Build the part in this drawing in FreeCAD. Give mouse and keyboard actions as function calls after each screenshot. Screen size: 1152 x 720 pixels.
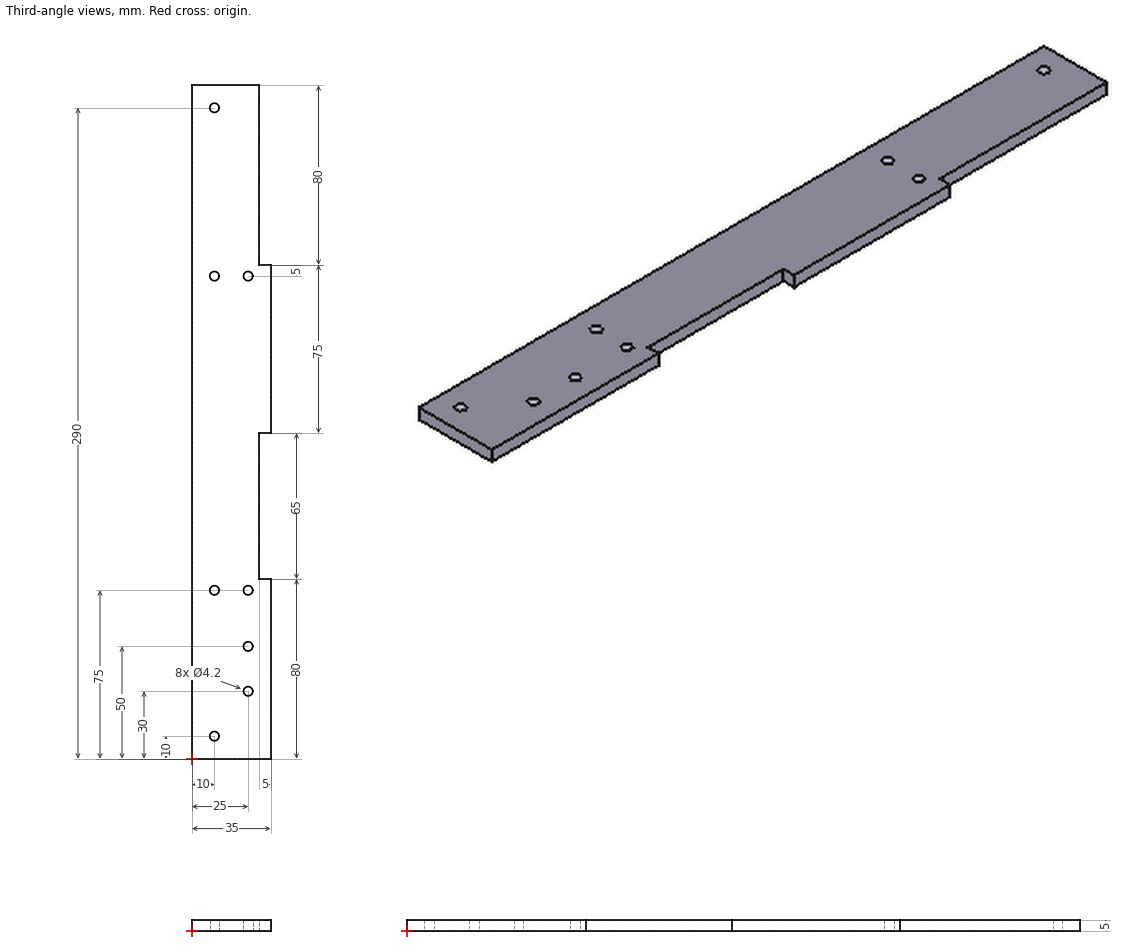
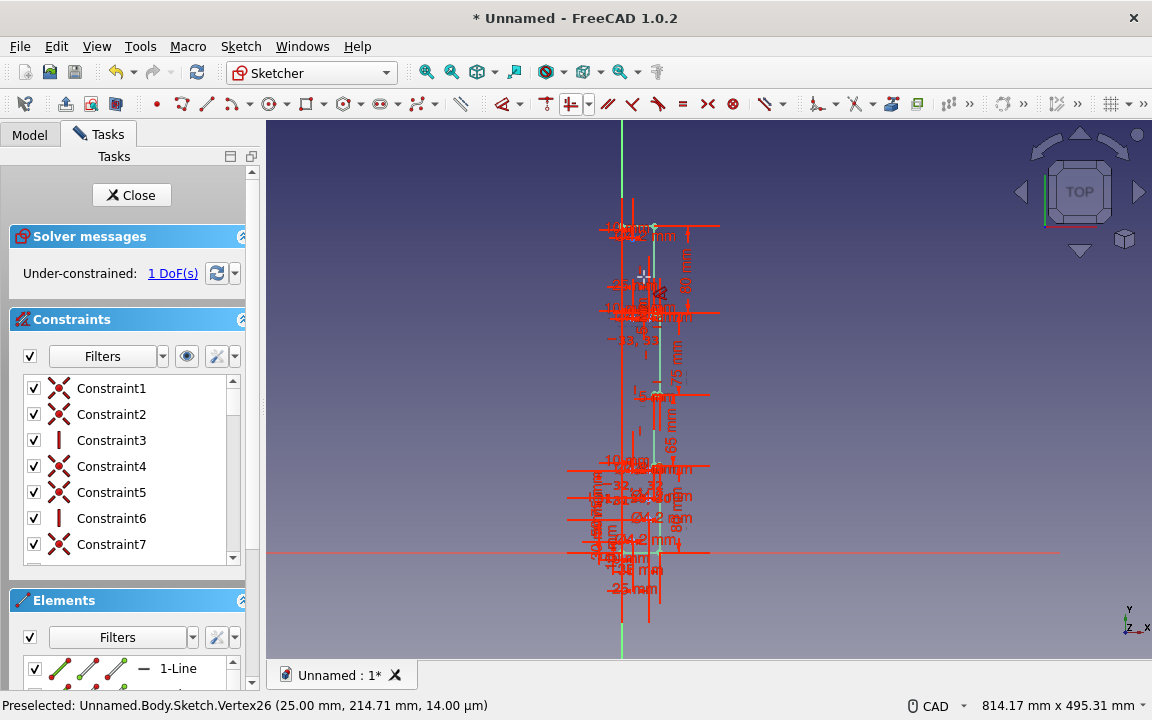
click(633, 238)
click(564, 395)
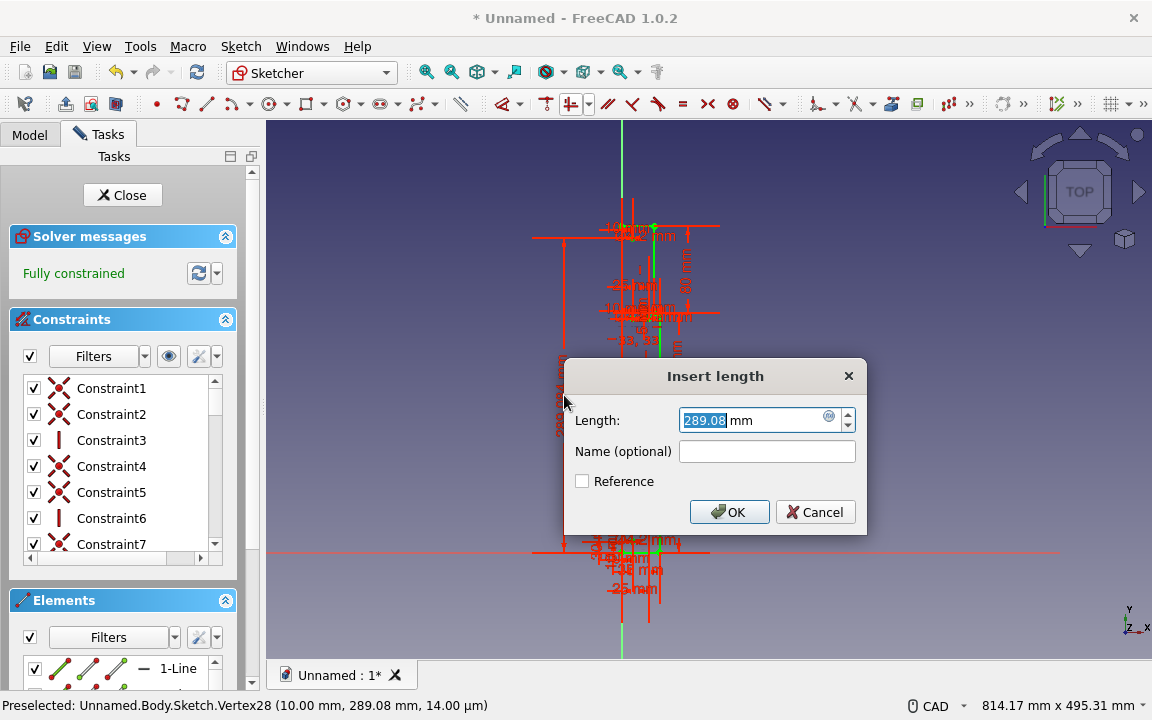
text(290)
key(Return)
key(Escape)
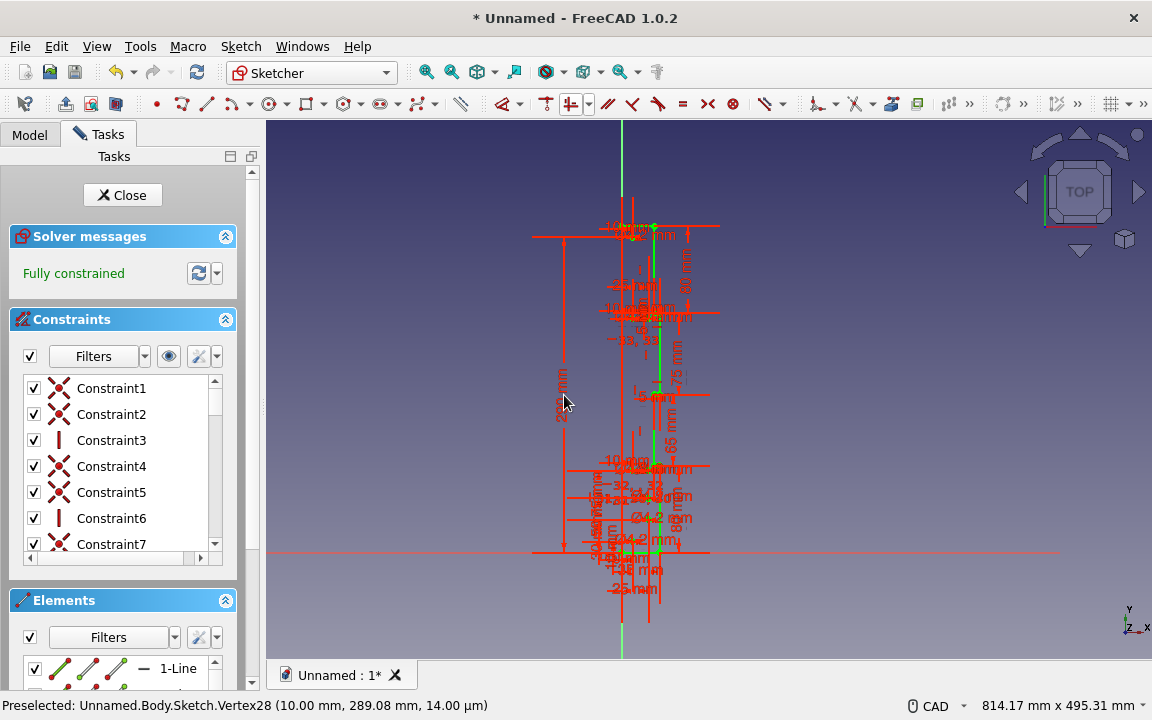
click(123, 195)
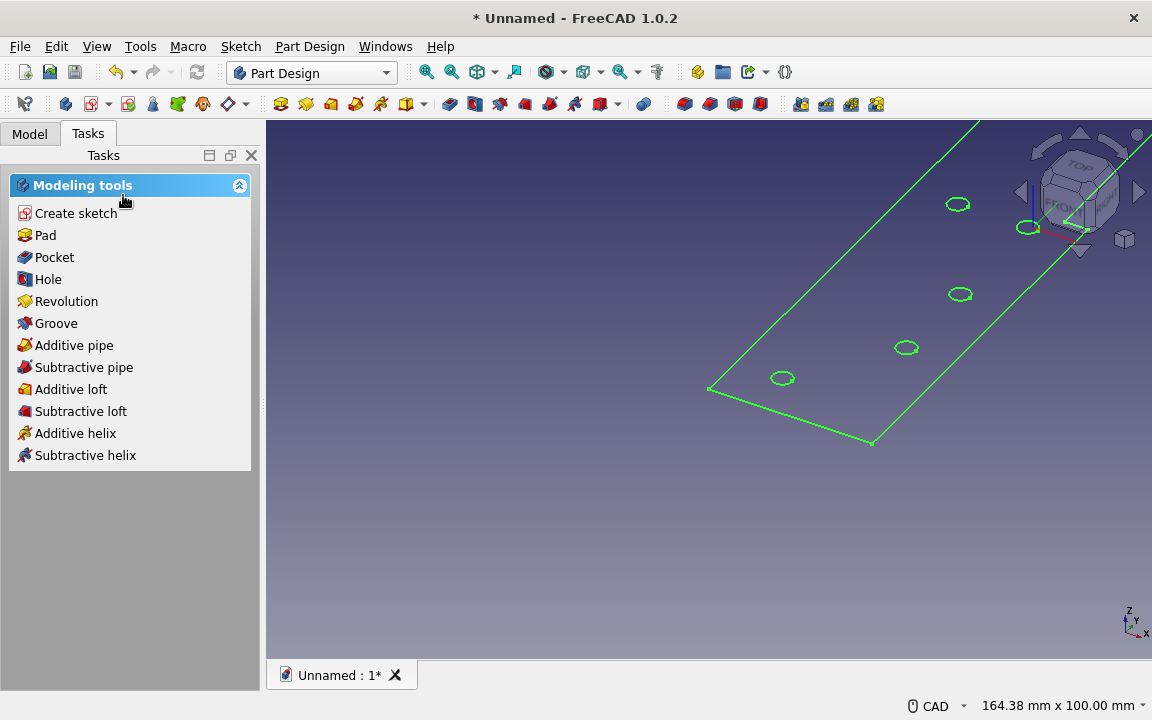
click(281, 104)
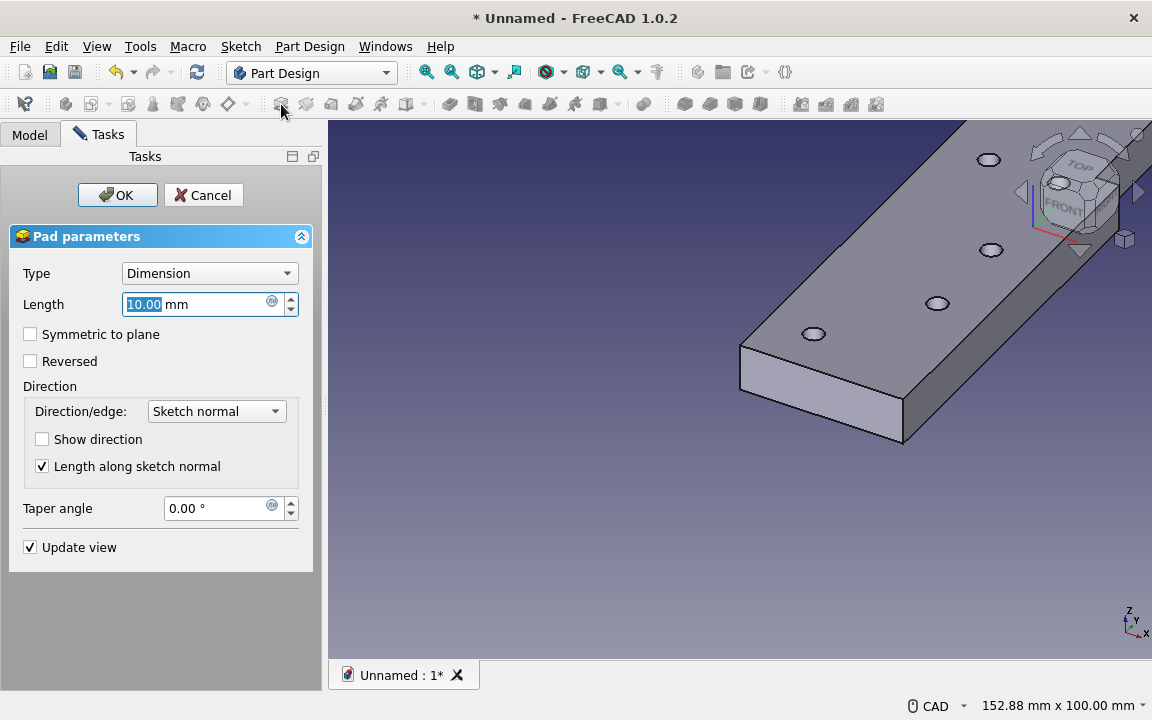
text(5)
key(Tab)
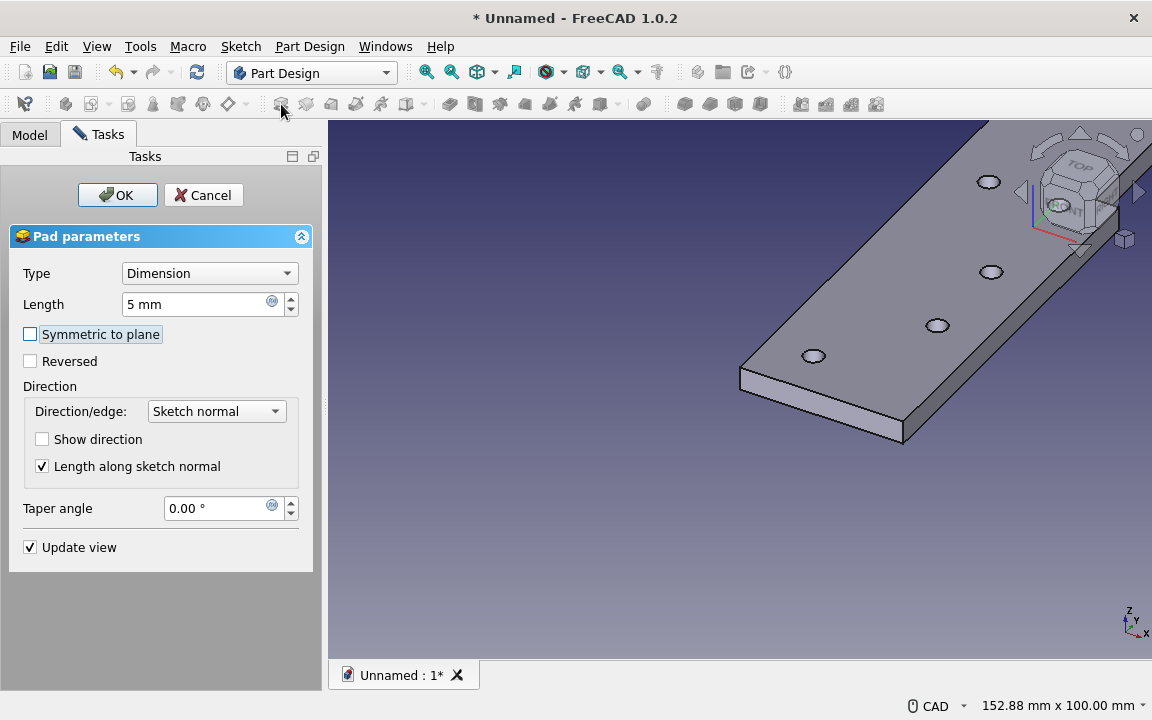
click(118, 195)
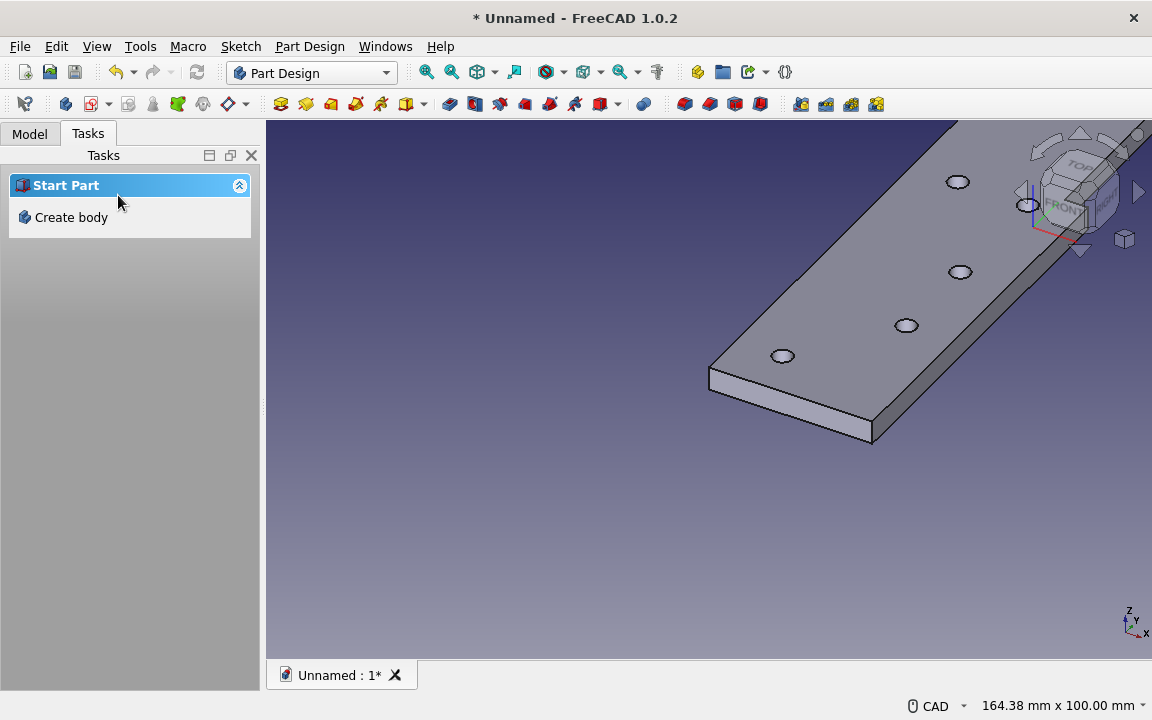
key(0)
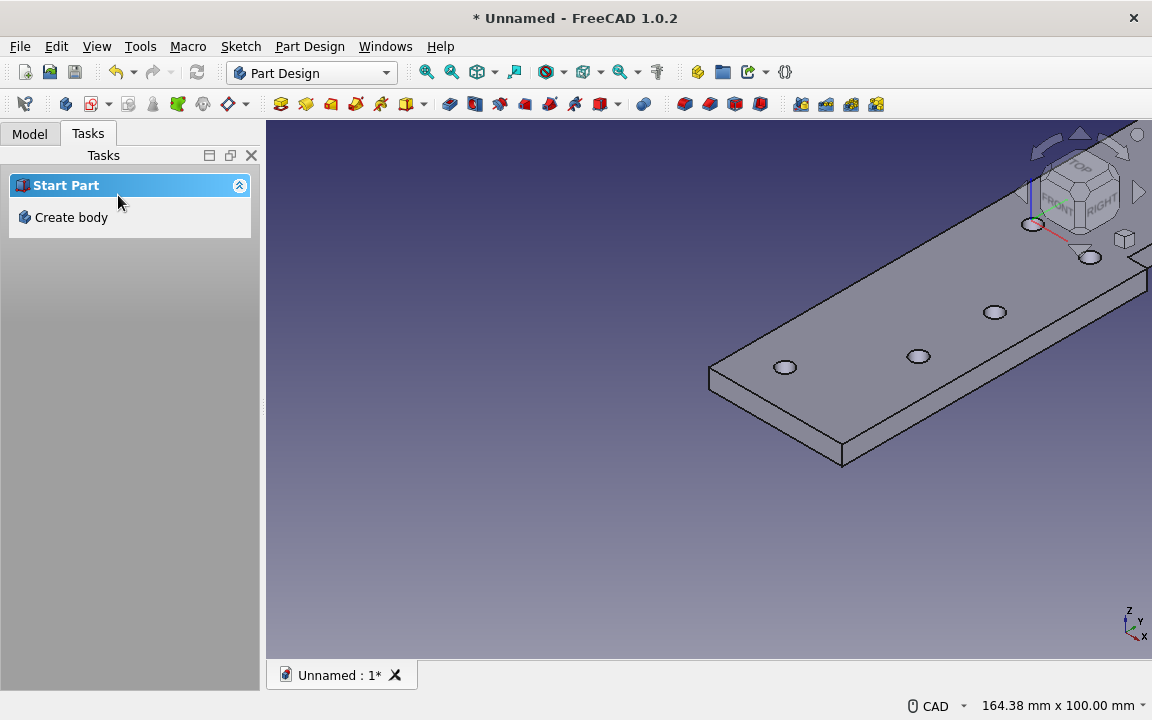
click(427, 72)